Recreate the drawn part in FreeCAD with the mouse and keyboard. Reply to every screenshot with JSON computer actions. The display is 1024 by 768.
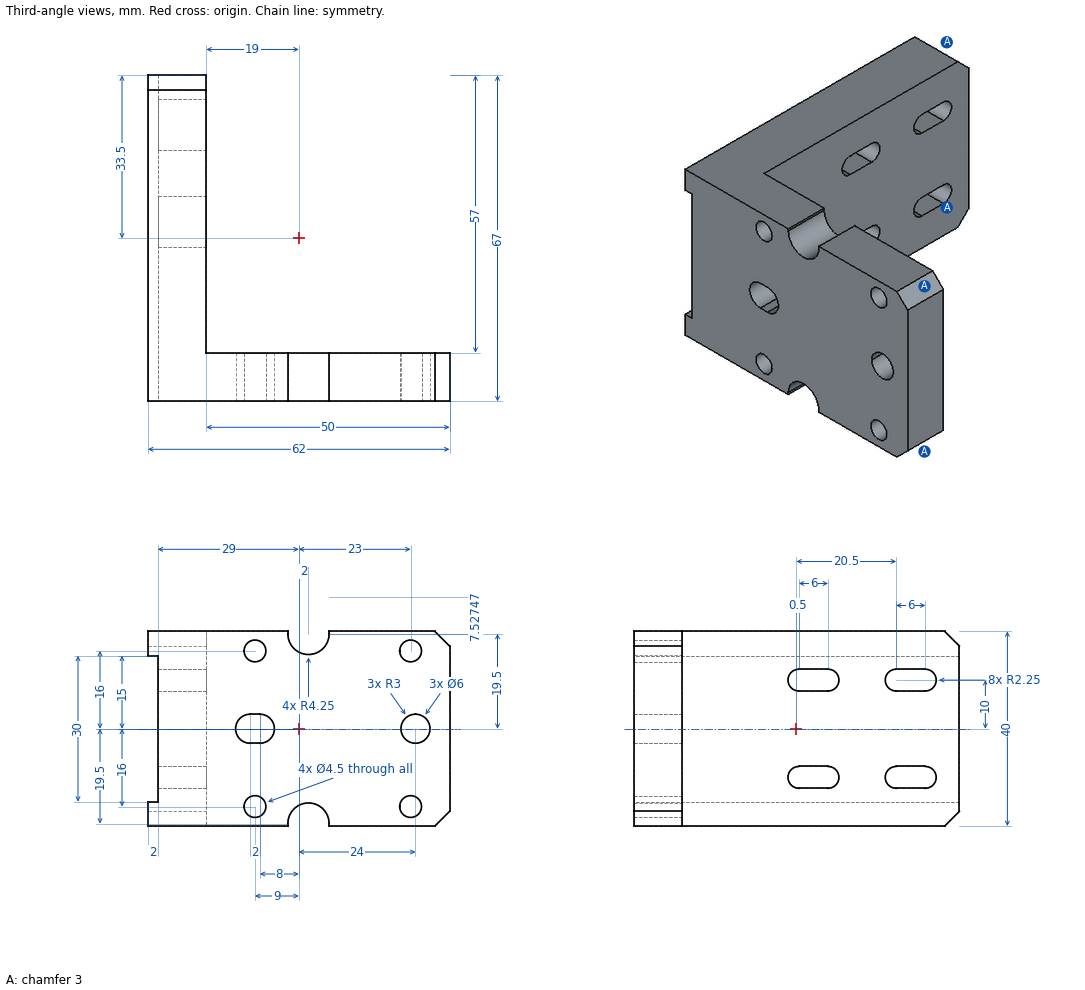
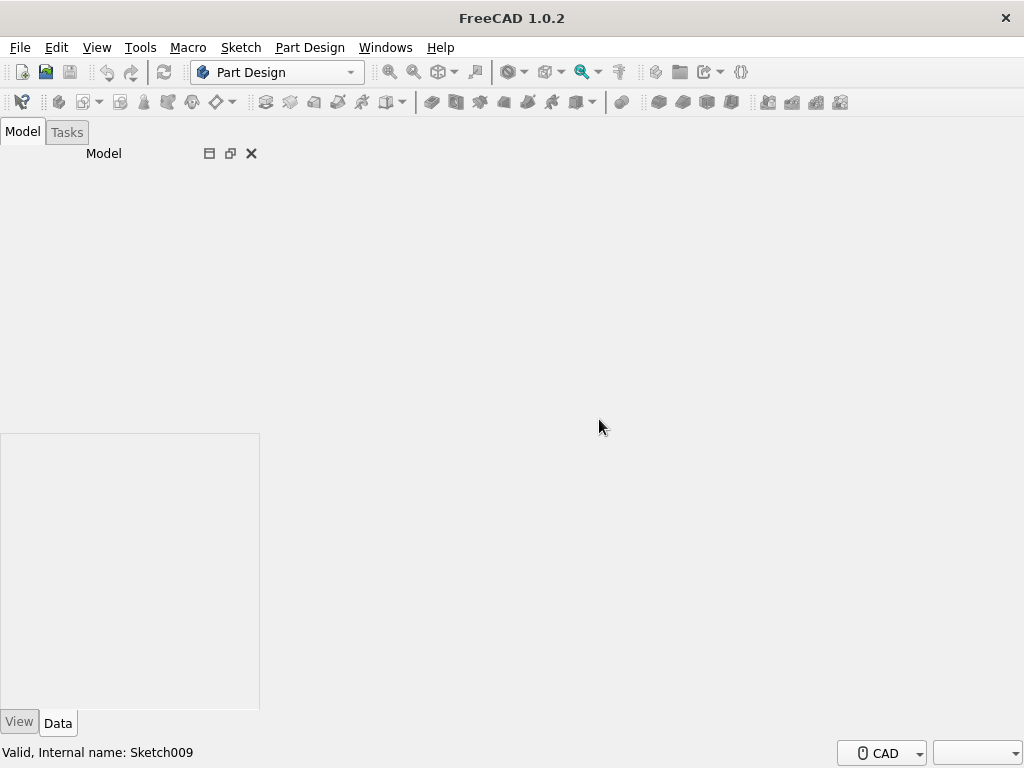
{"action": "left_click", "coordinate": [22, 72]}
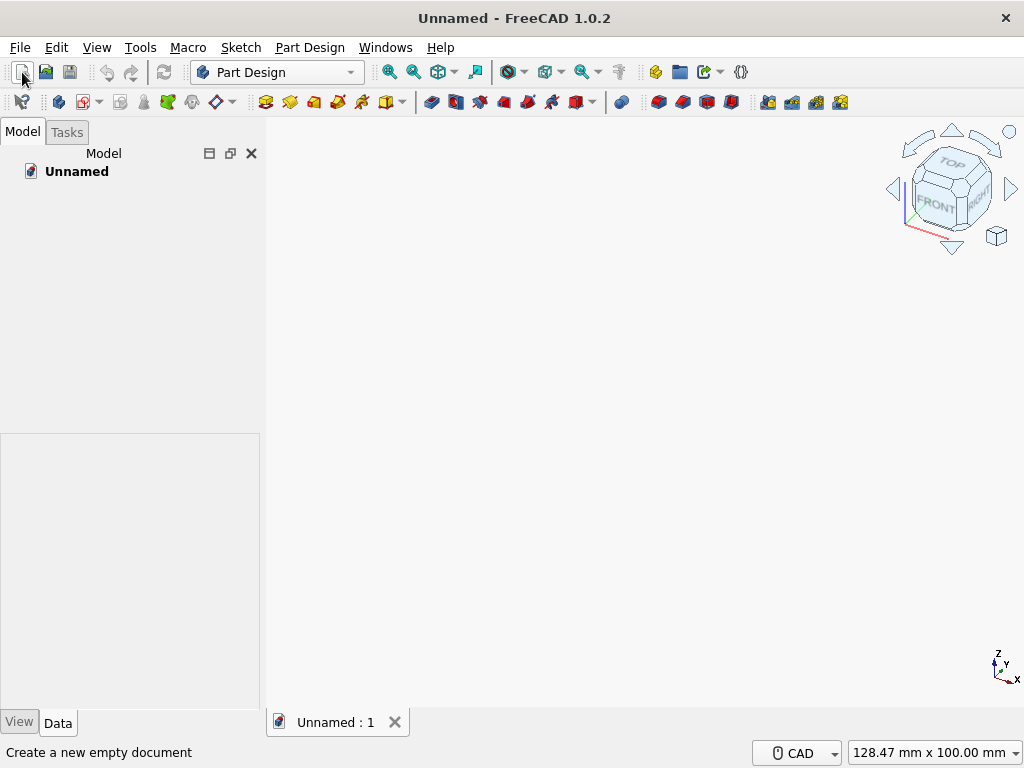
{"action": "left_click", "coordinate": [84, 102]}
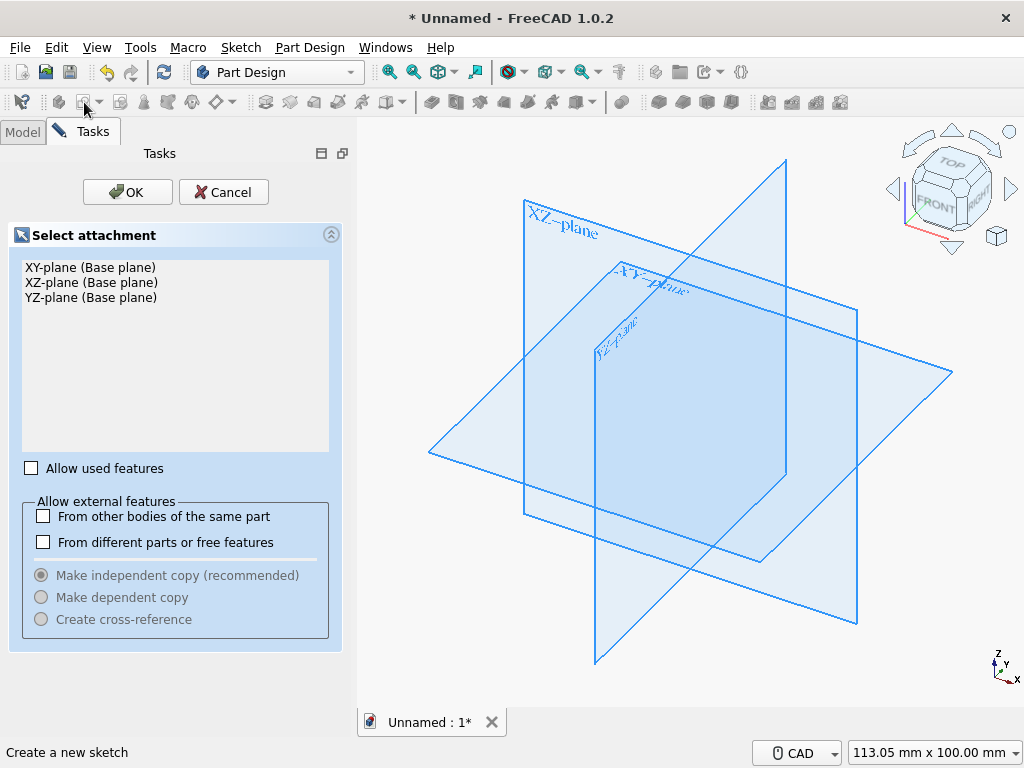
{"action": "left_click", "coordinate": [82, 268]}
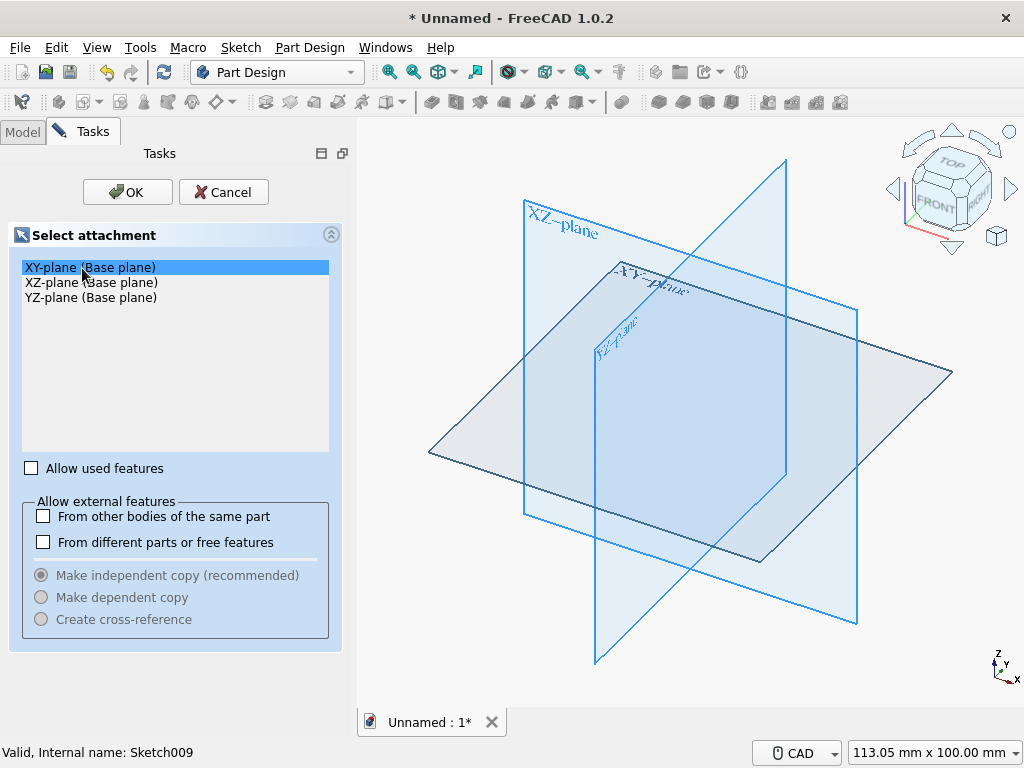
{"action": "left_click", "coordinate": [128, 192]}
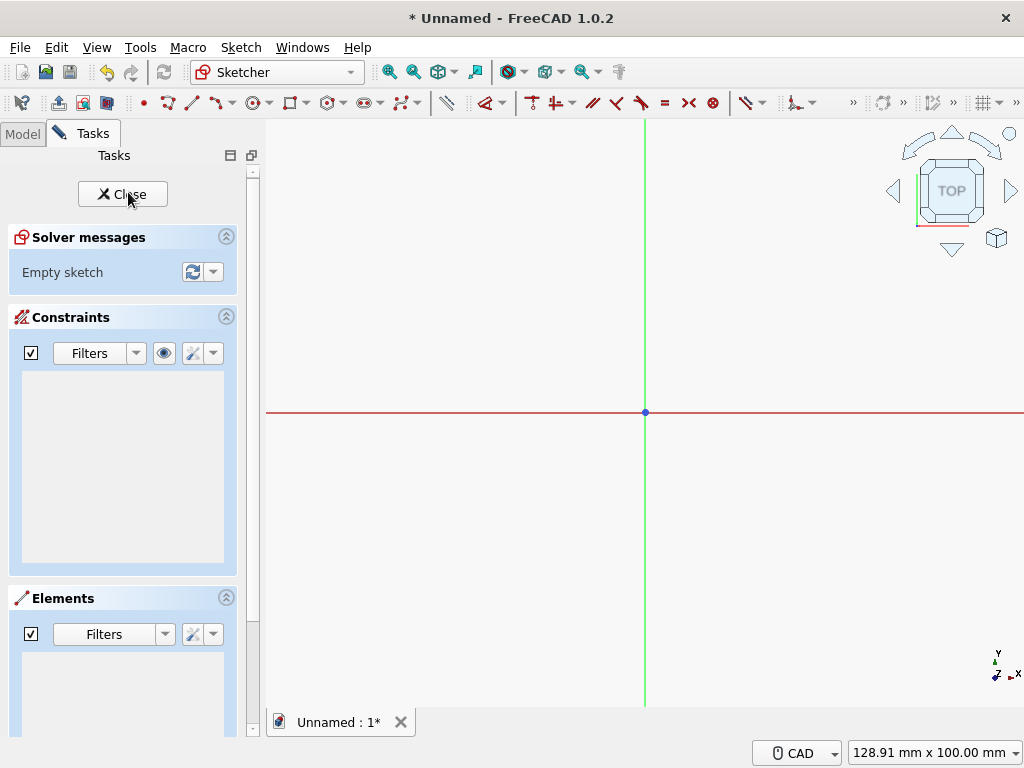
{"action": "left_click", "coordinate": [308, 104]}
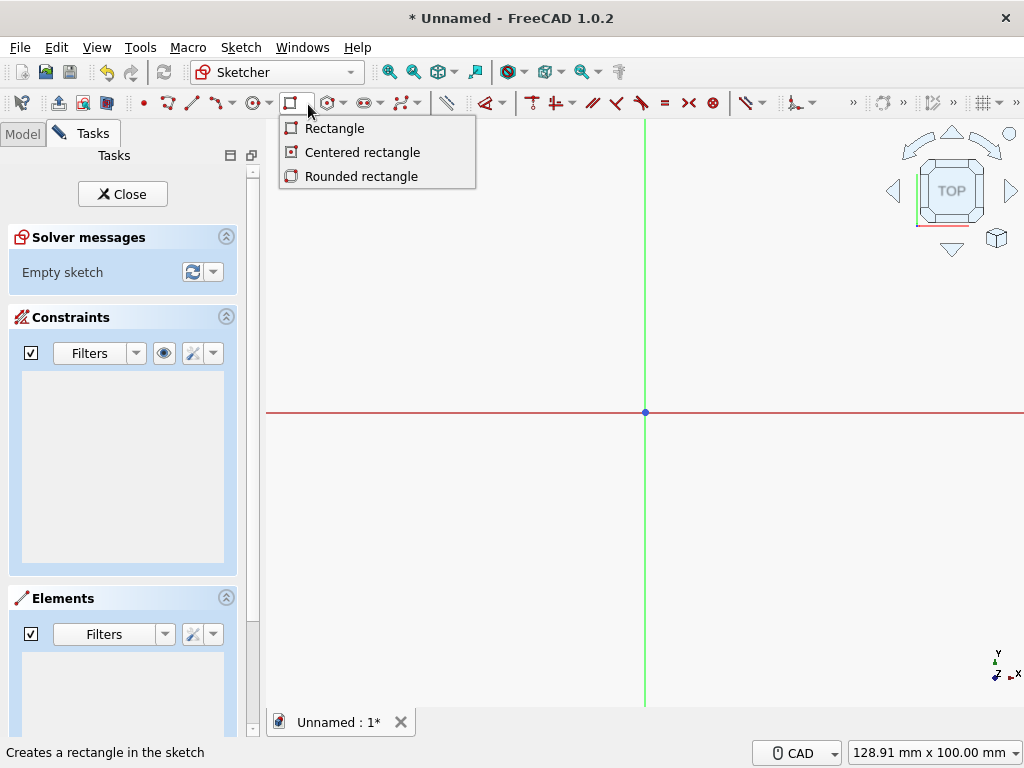
{"action": "left_click", "coordinate": [378, 152]}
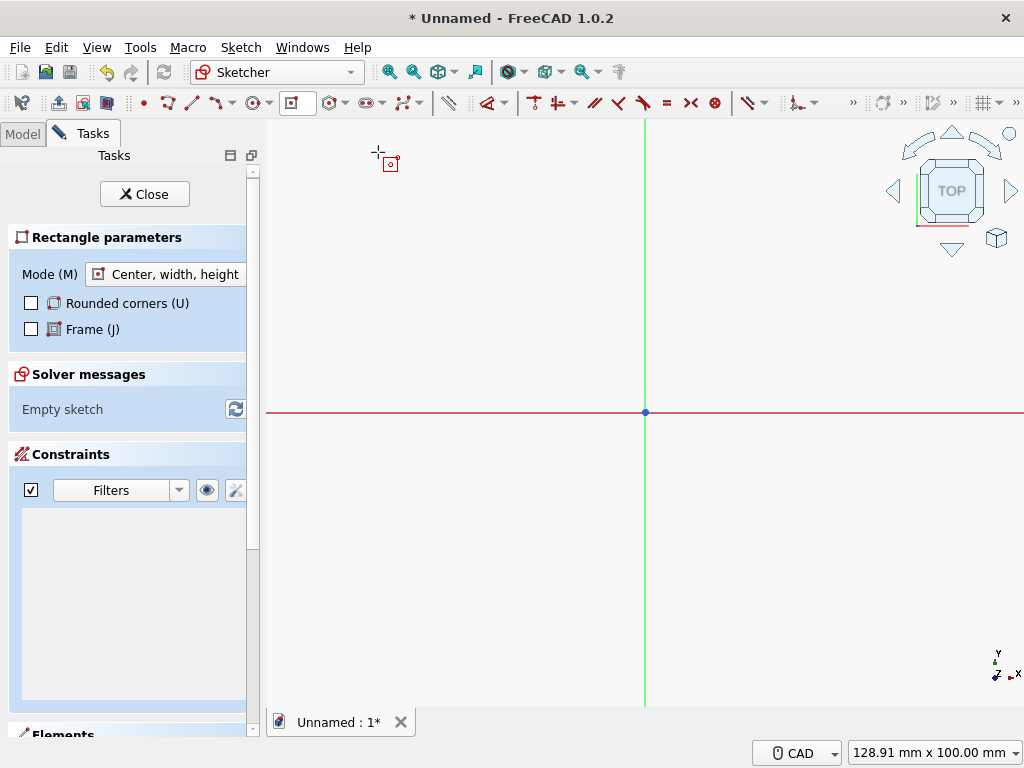
{"action": "left_click", "coordinate": [645, 413]}
{"action": "mouse_move", "coordinate": [827, 216]}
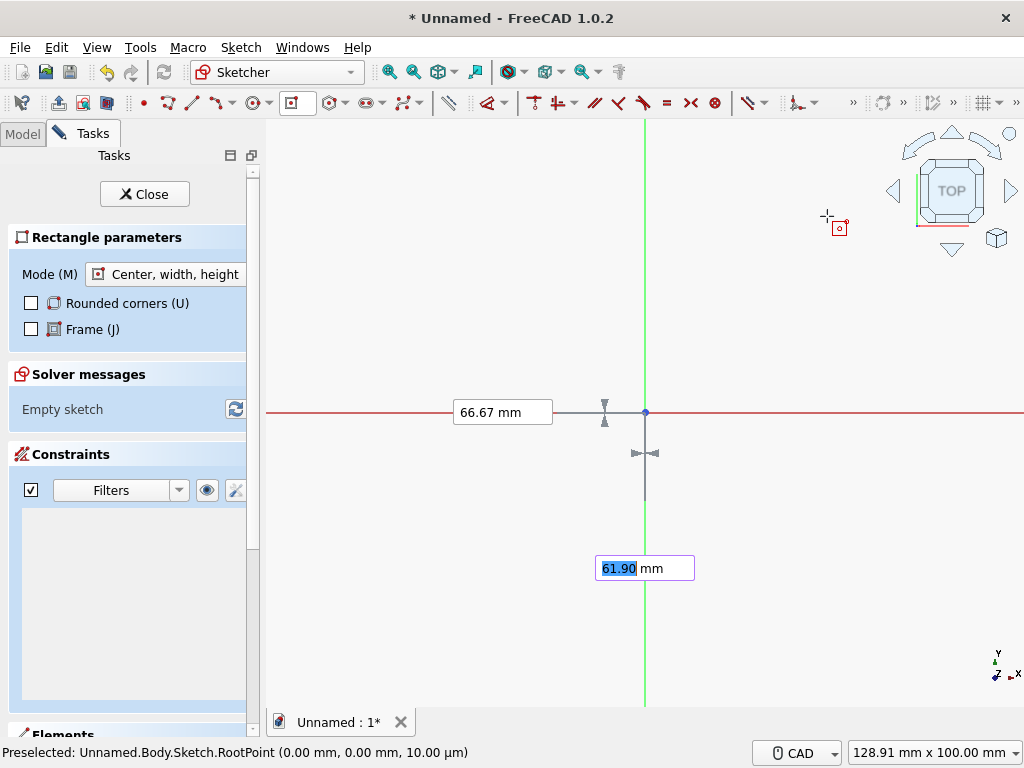
{"action": "type", "text": "62"}
{"action": "key", "text": "Tab"}
{"action": "type", "text": "67"}
{"action": "key", "text": "Return"}
{"action": "key", "text": "Escape"}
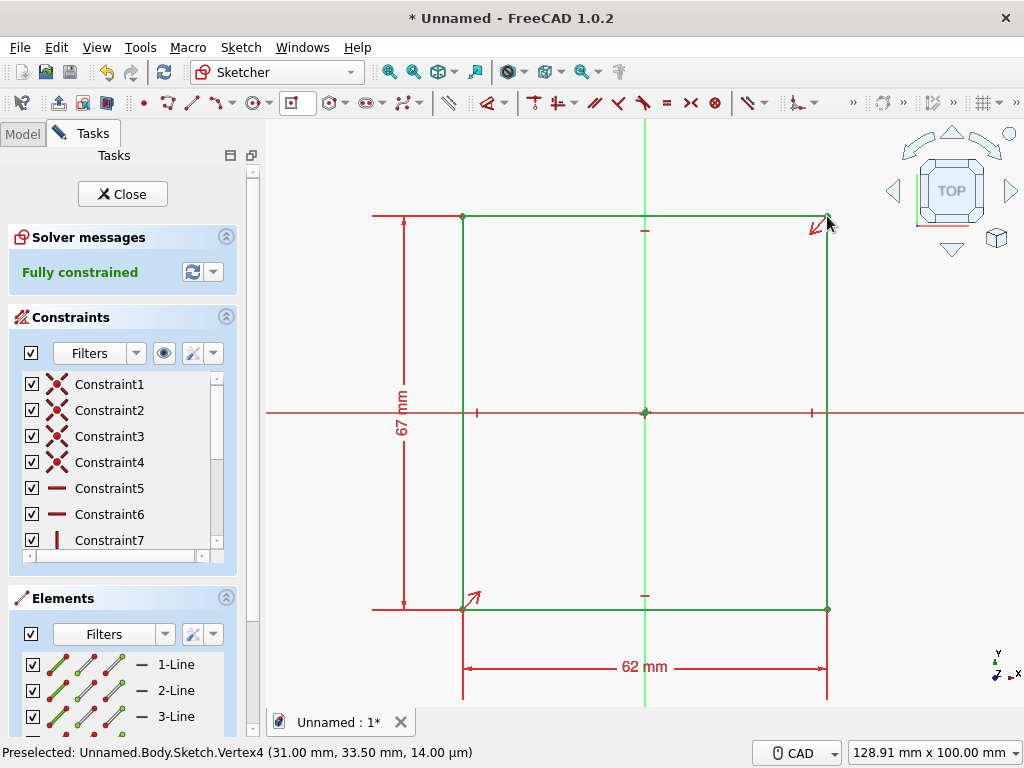
{"action": "left_click", "coordinate": [123, 194]}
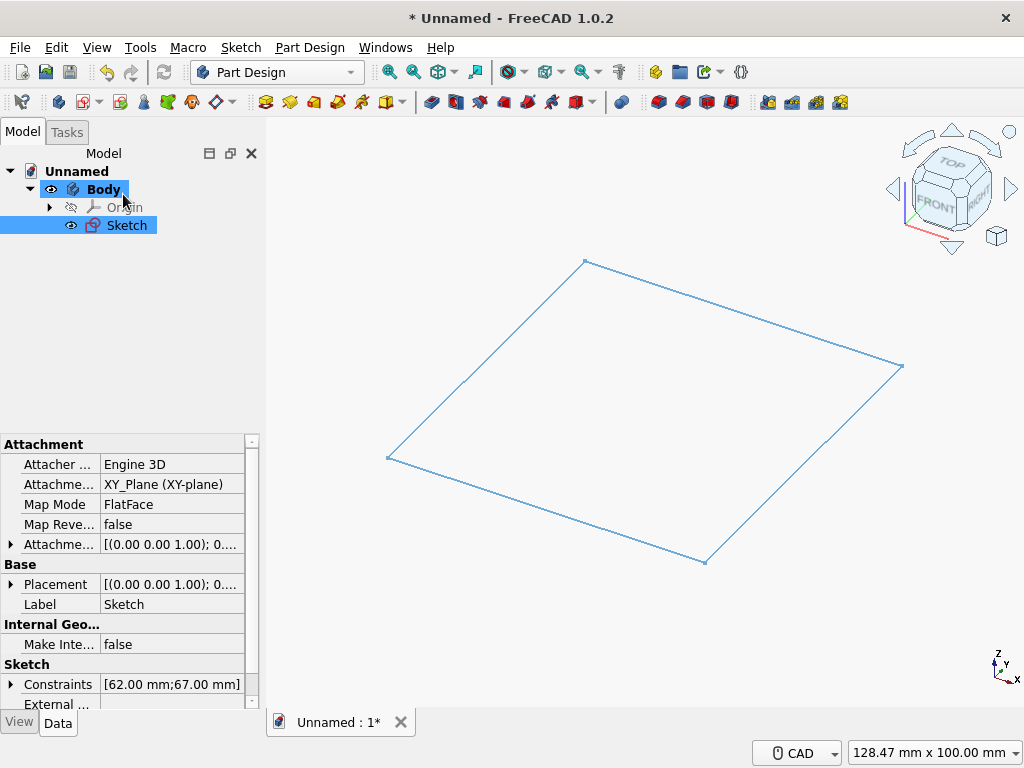
{"action": "left_click", "coordinate": [266, 102]}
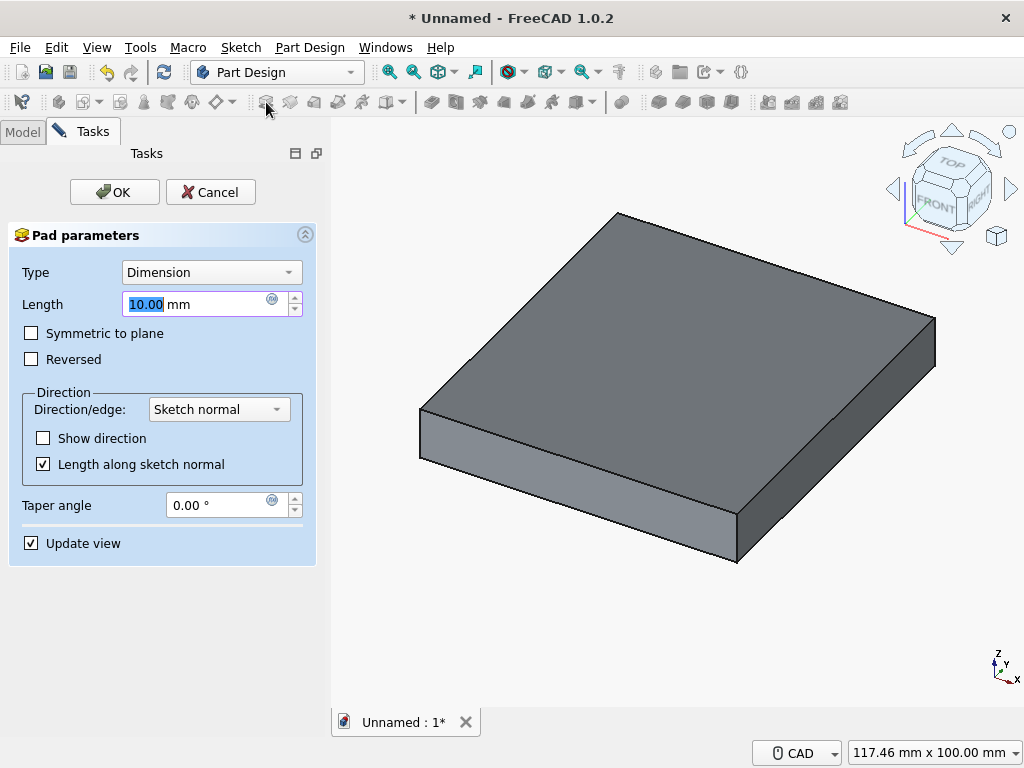
{"action": "type", "text": "40"}
{"action": "key", "text": "Tab"}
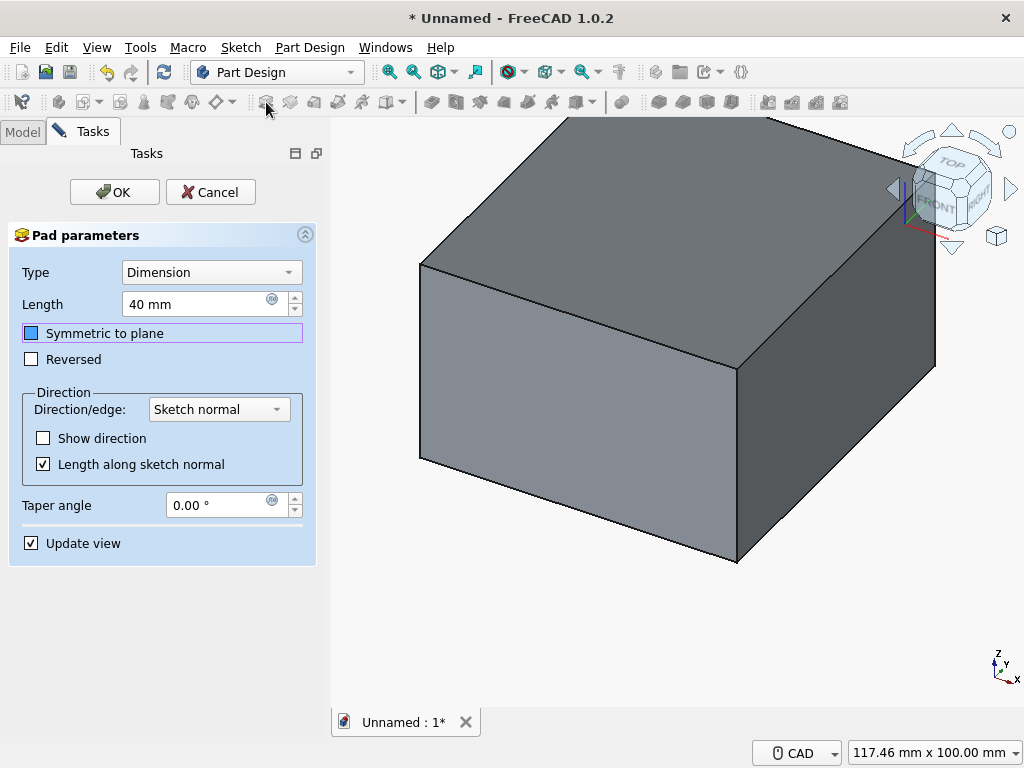
{"action": "left_click", "coordinate": [30, 333]}